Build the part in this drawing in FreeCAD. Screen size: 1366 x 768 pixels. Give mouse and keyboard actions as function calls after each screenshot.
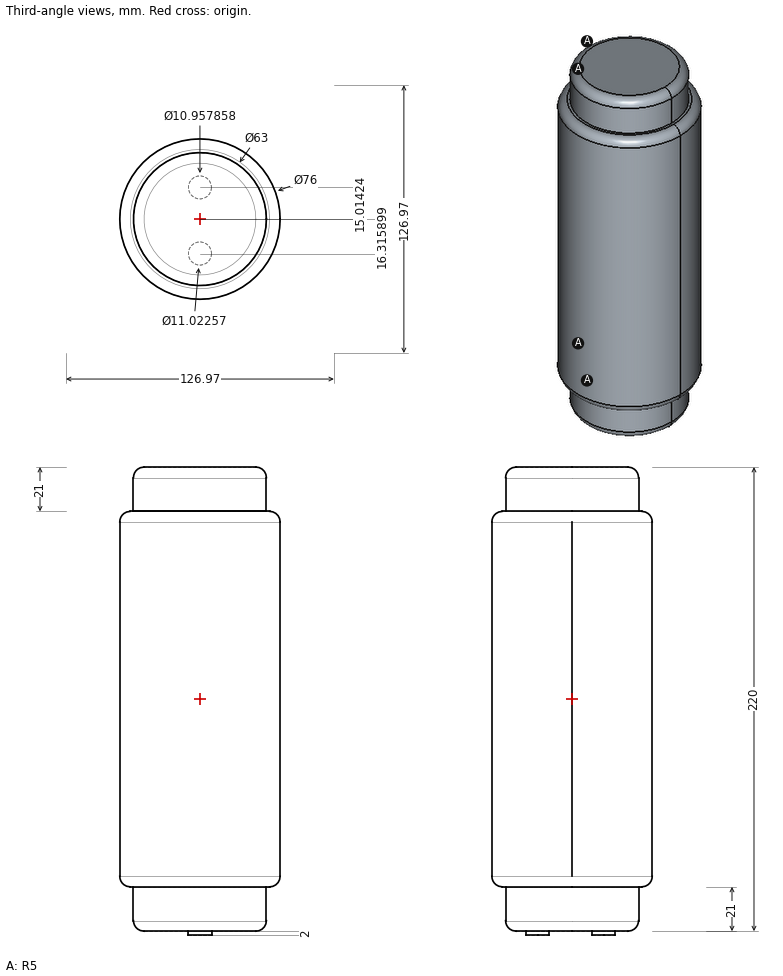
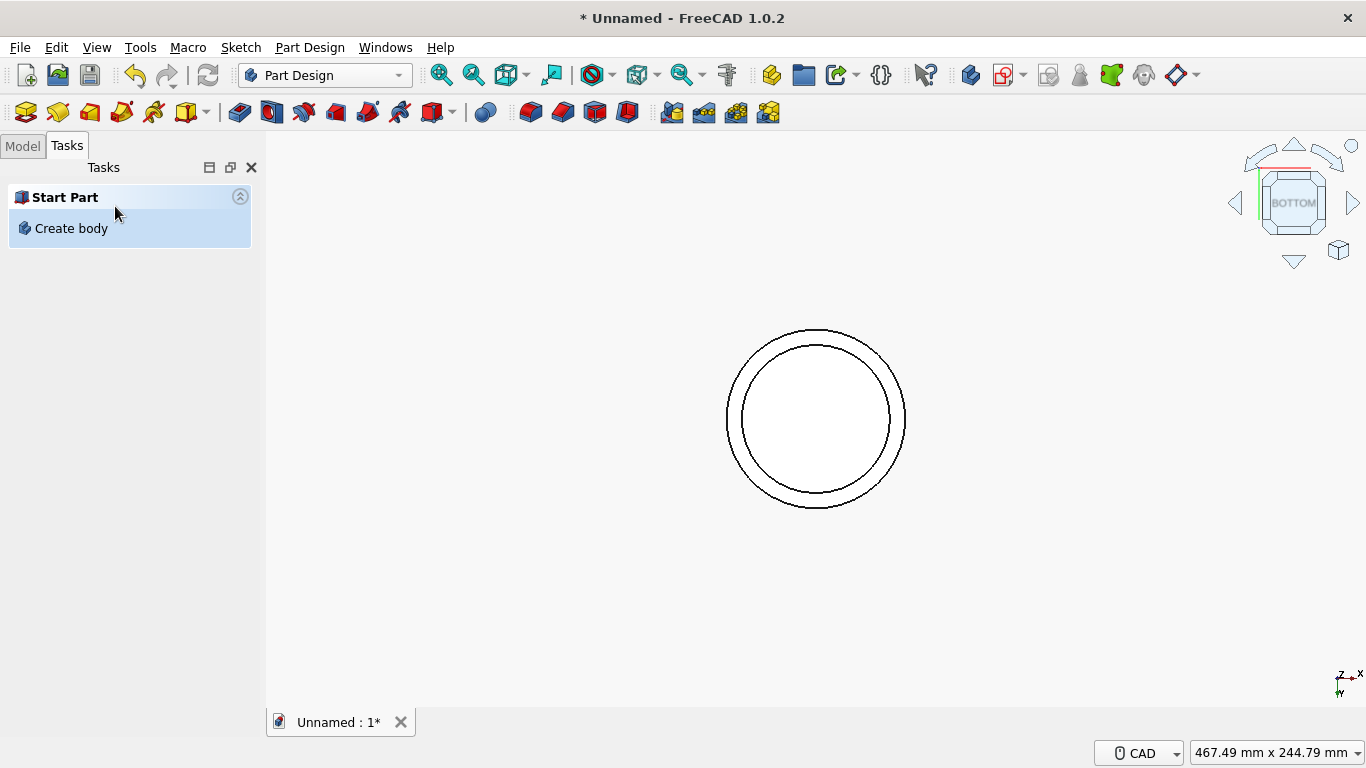
key(v)
key(f)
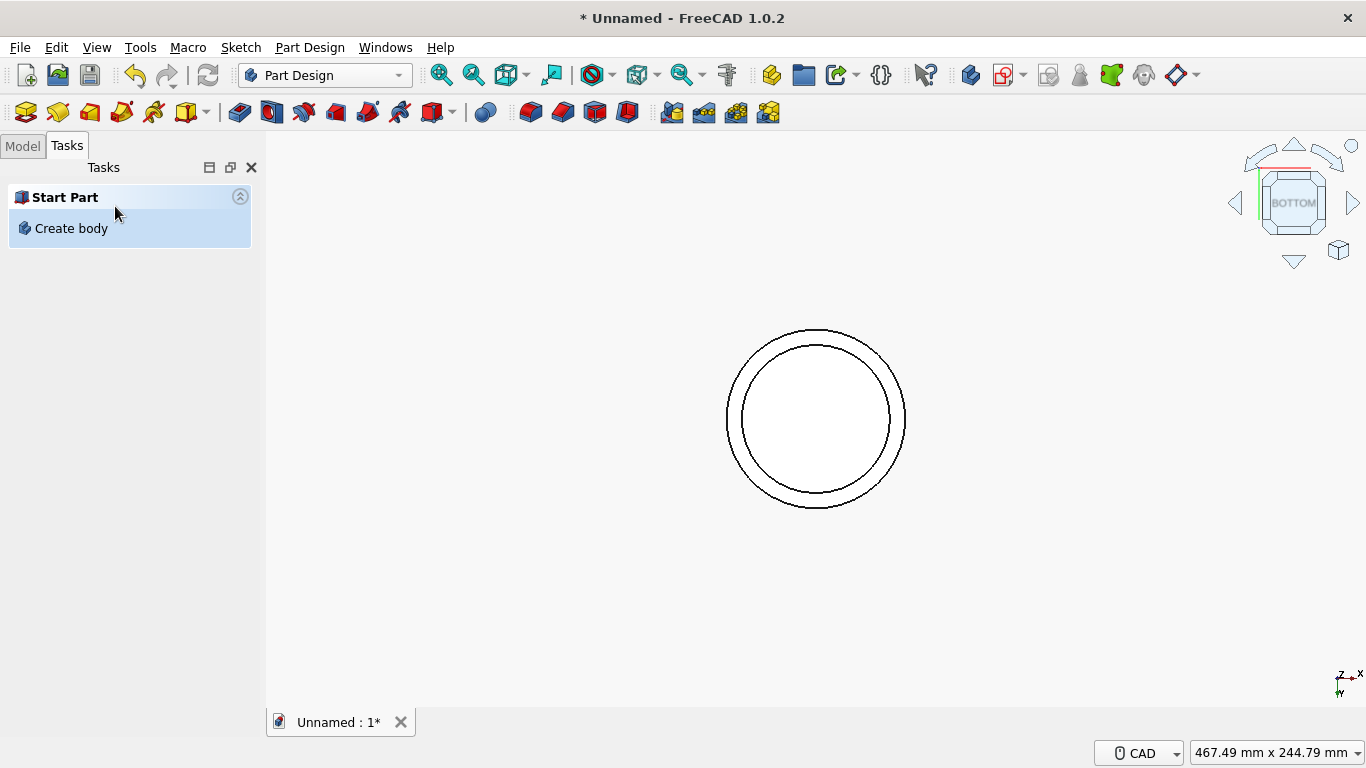
click(726, 418)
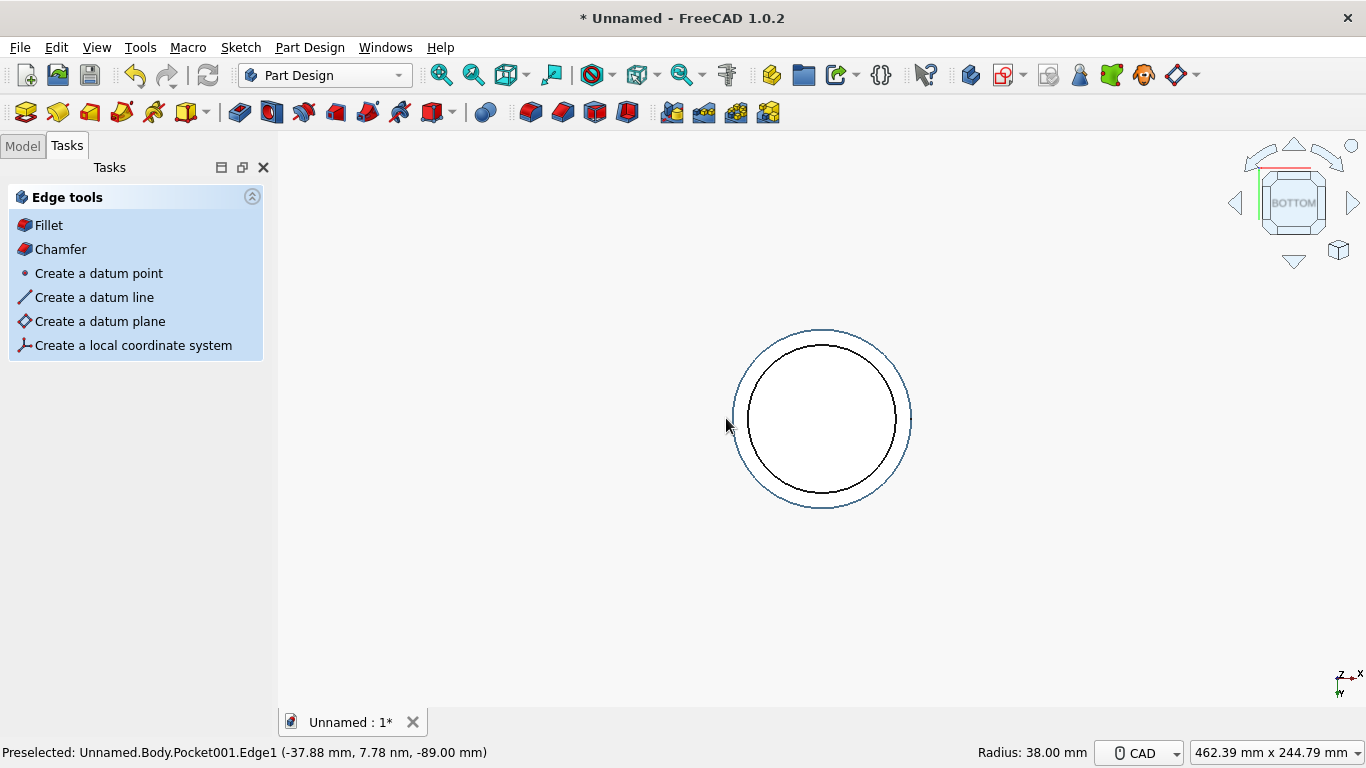
click(748, 418, ctrl)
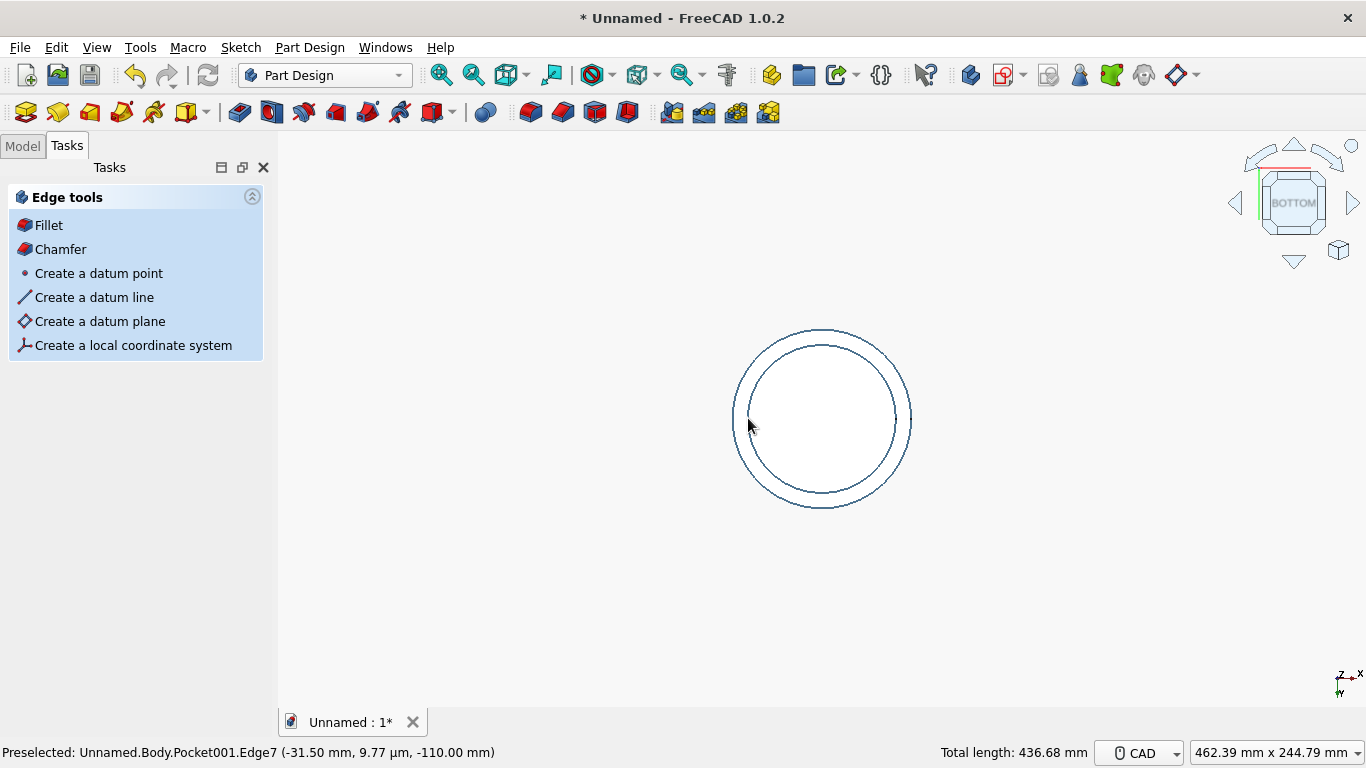
key(0)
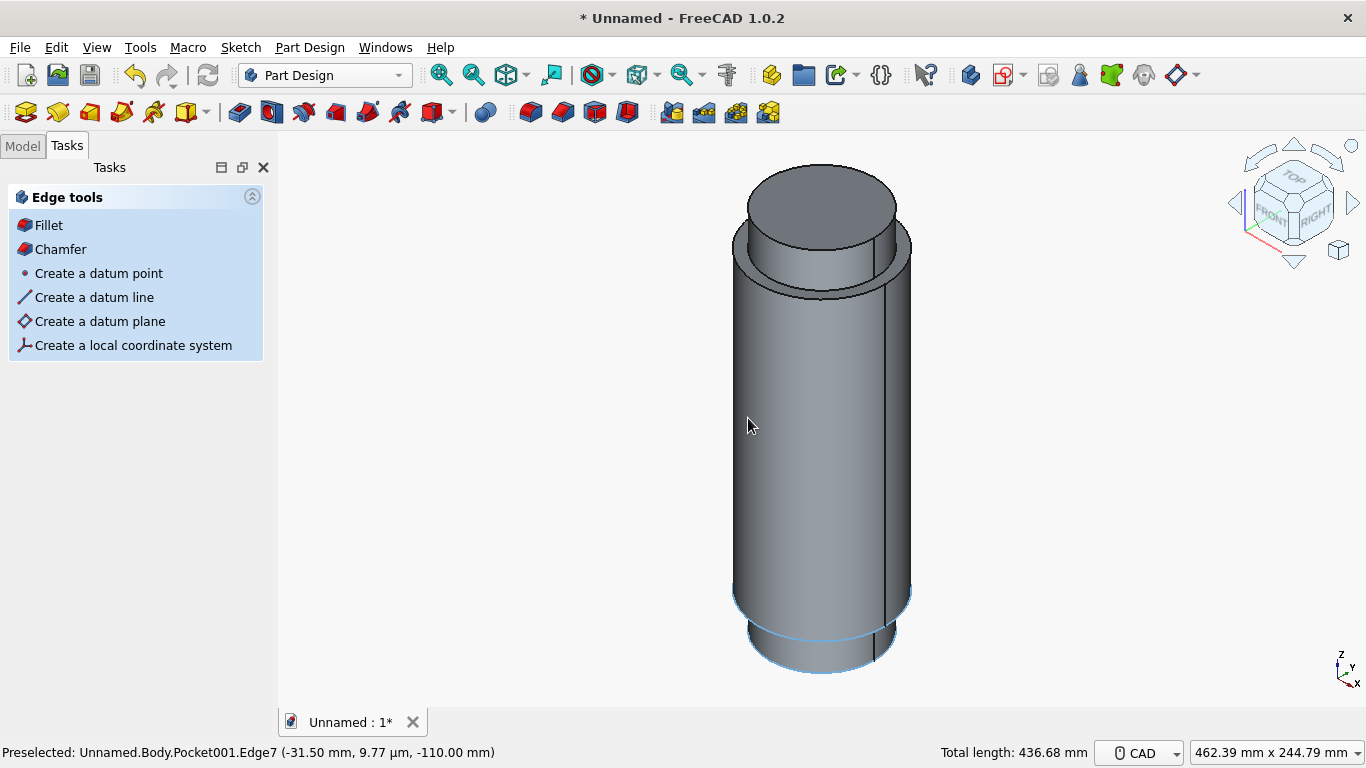
click(756, 226, ctrl)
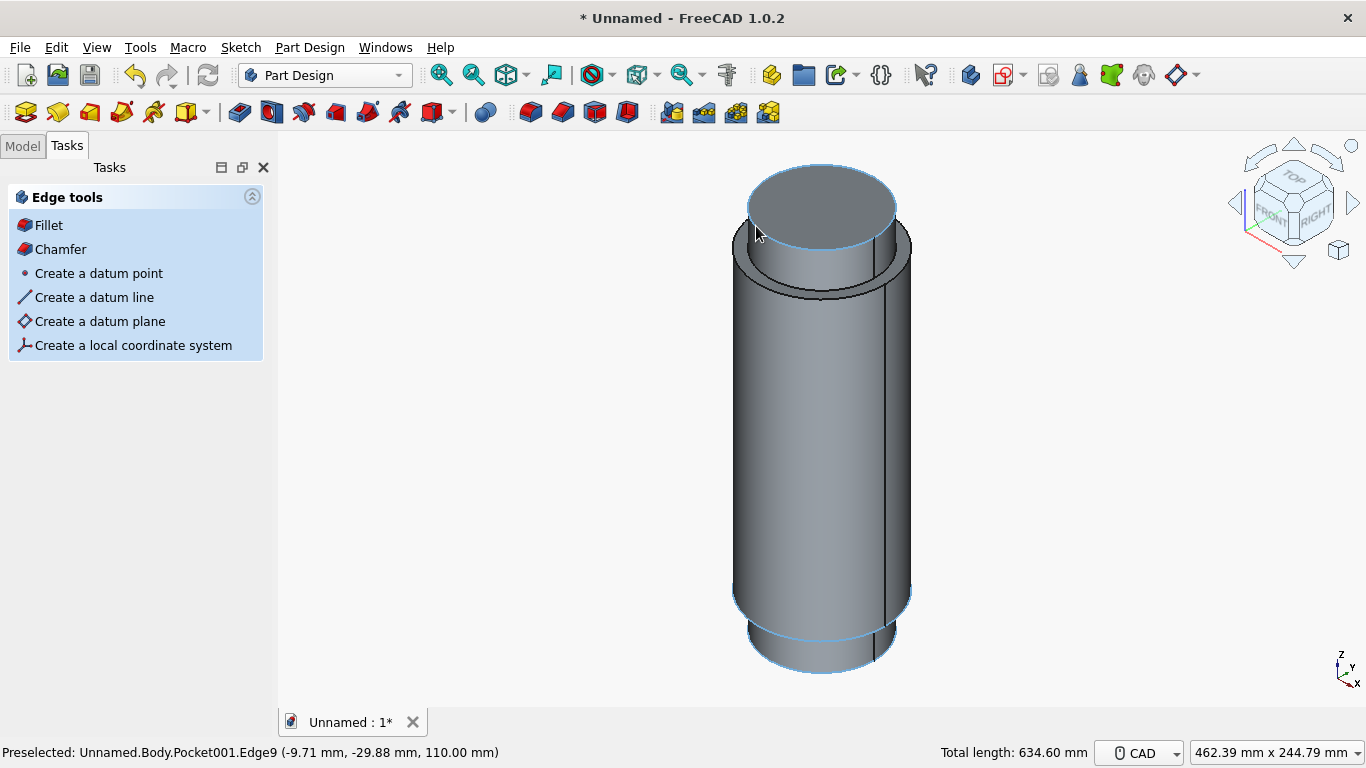
click(742, 270, ctrl)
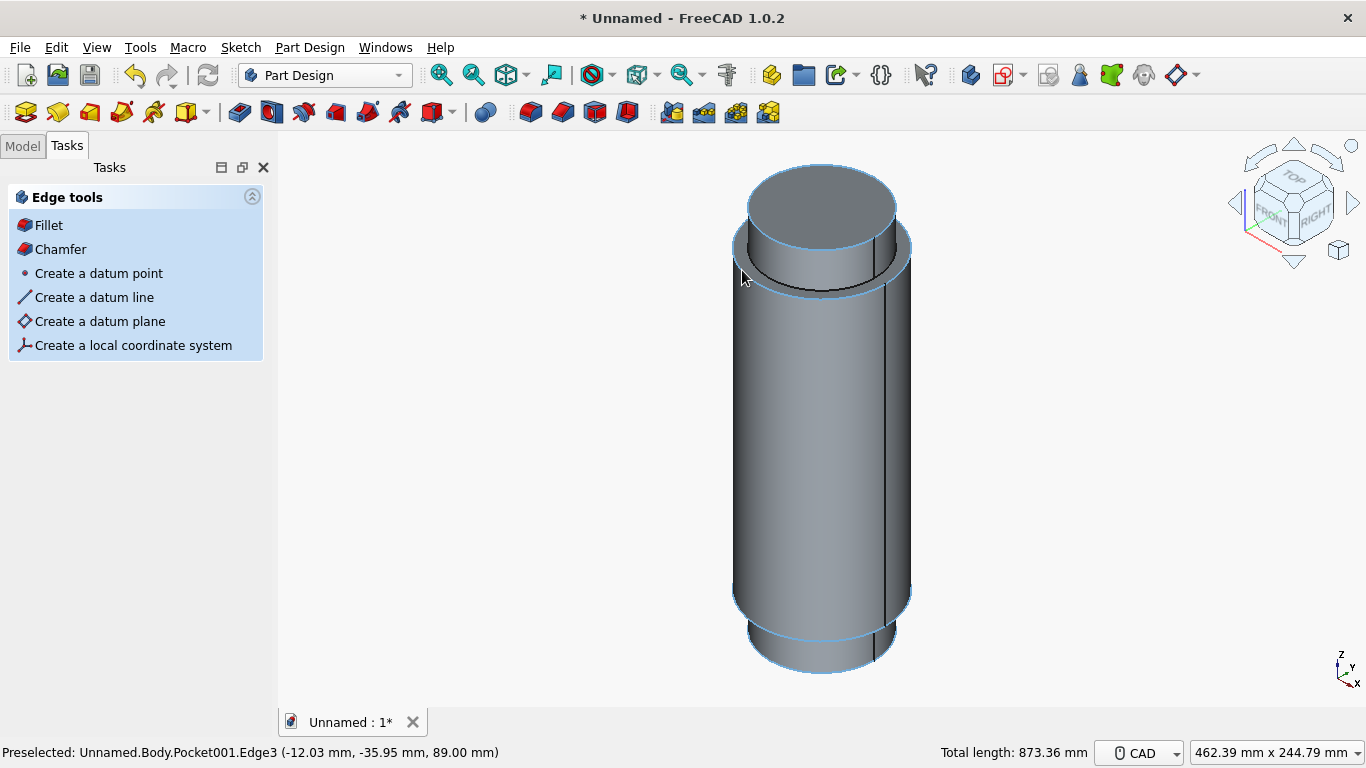
click(532, 112)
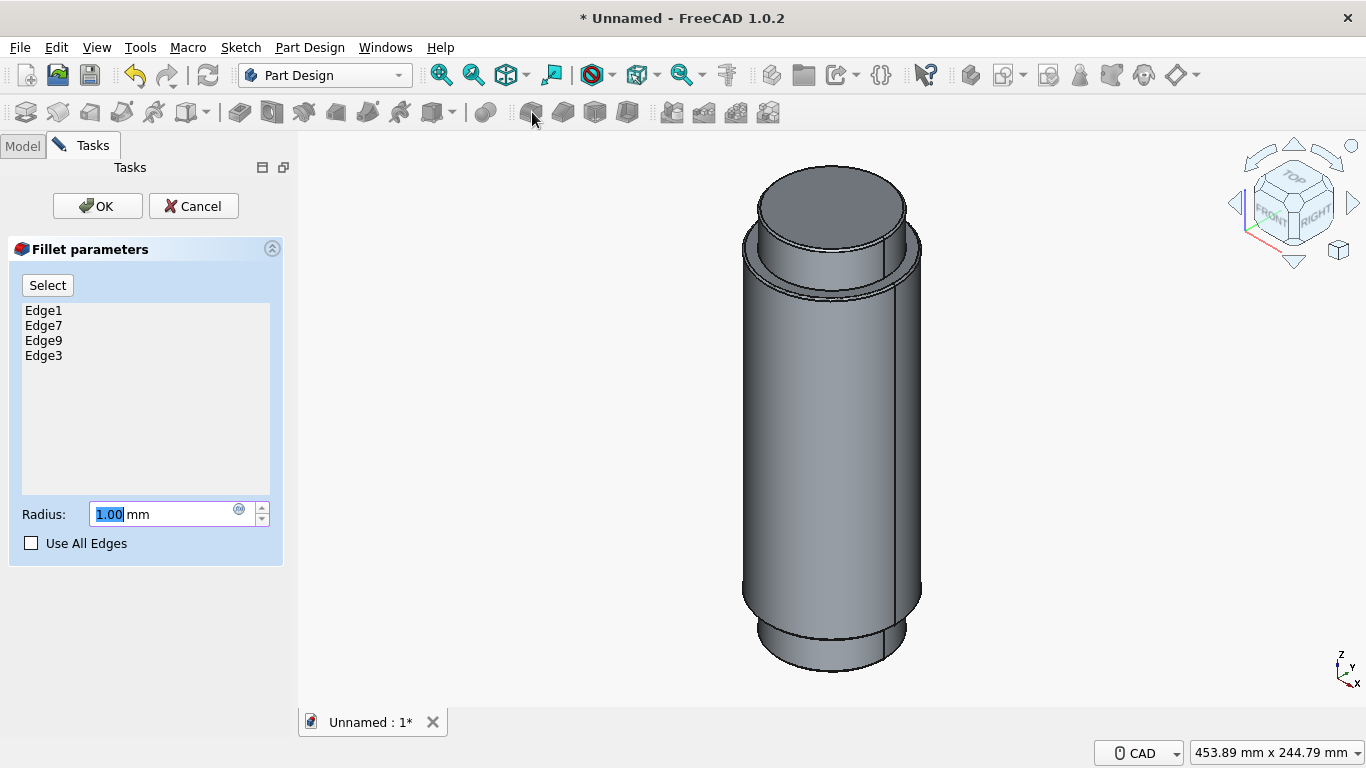
text(5)
key(Tab)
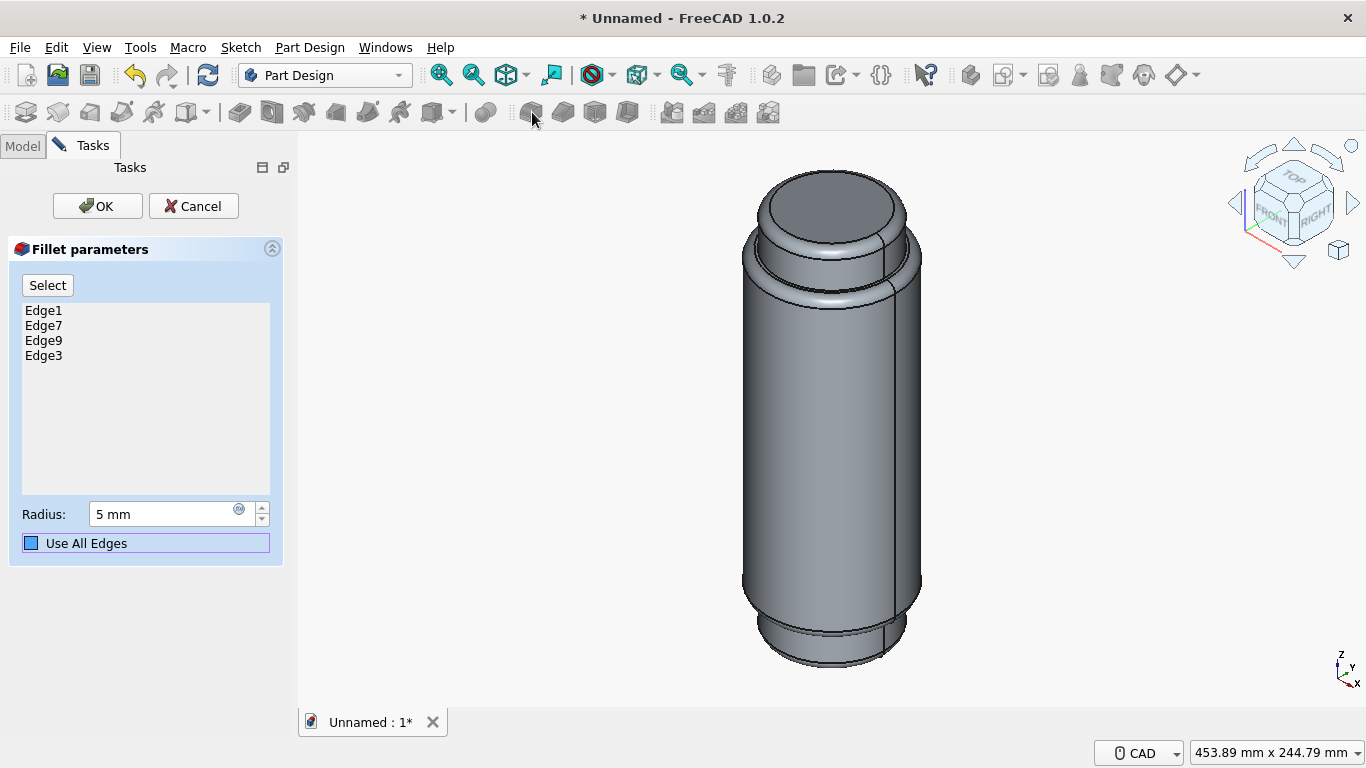
click(98, 206)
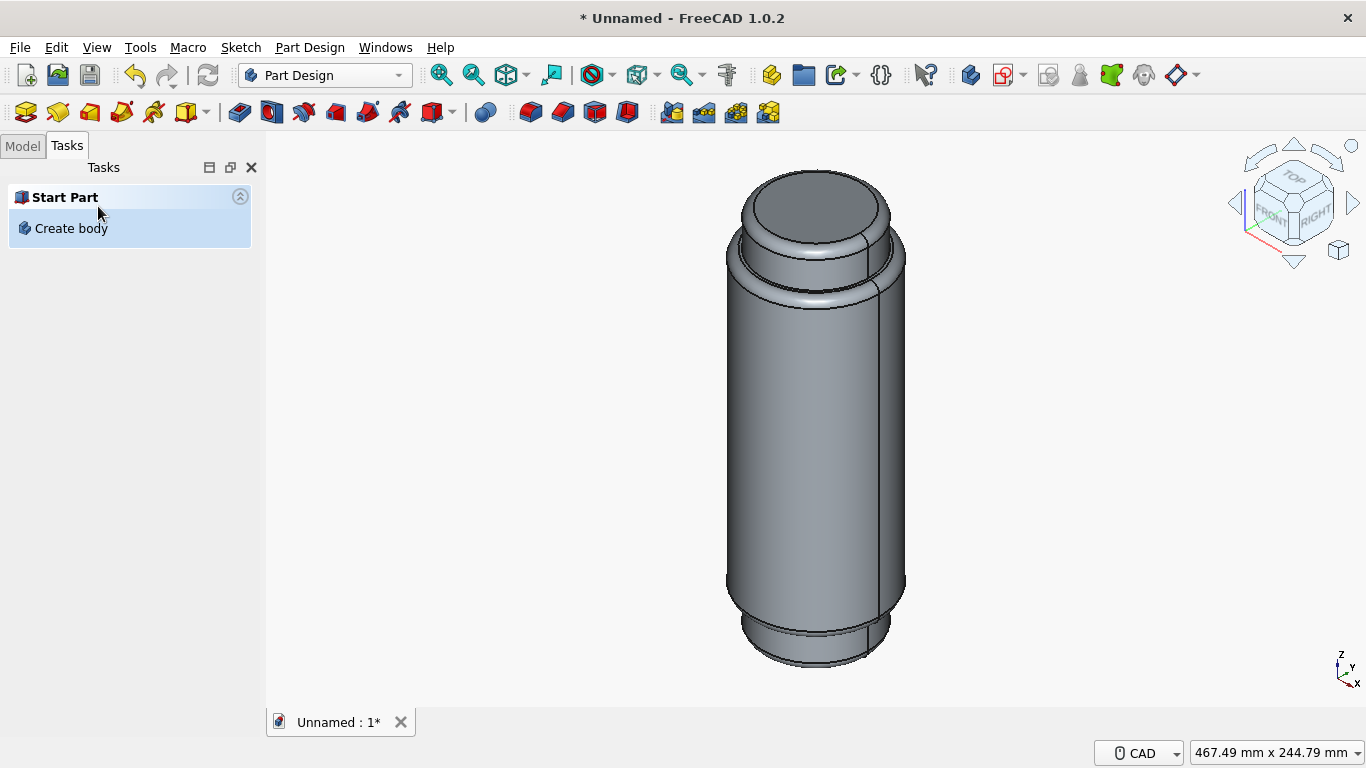
key(5)